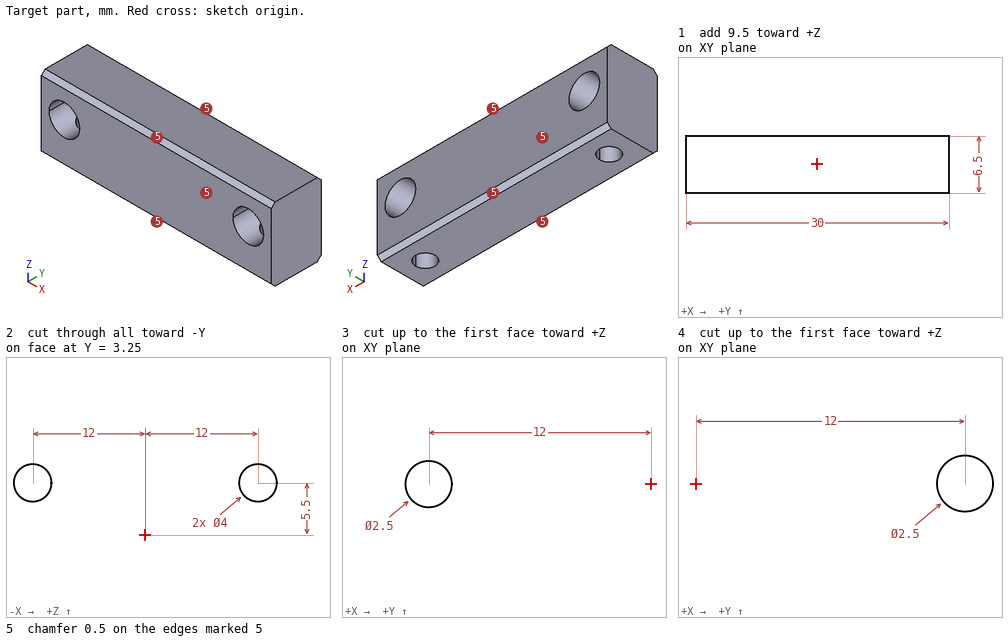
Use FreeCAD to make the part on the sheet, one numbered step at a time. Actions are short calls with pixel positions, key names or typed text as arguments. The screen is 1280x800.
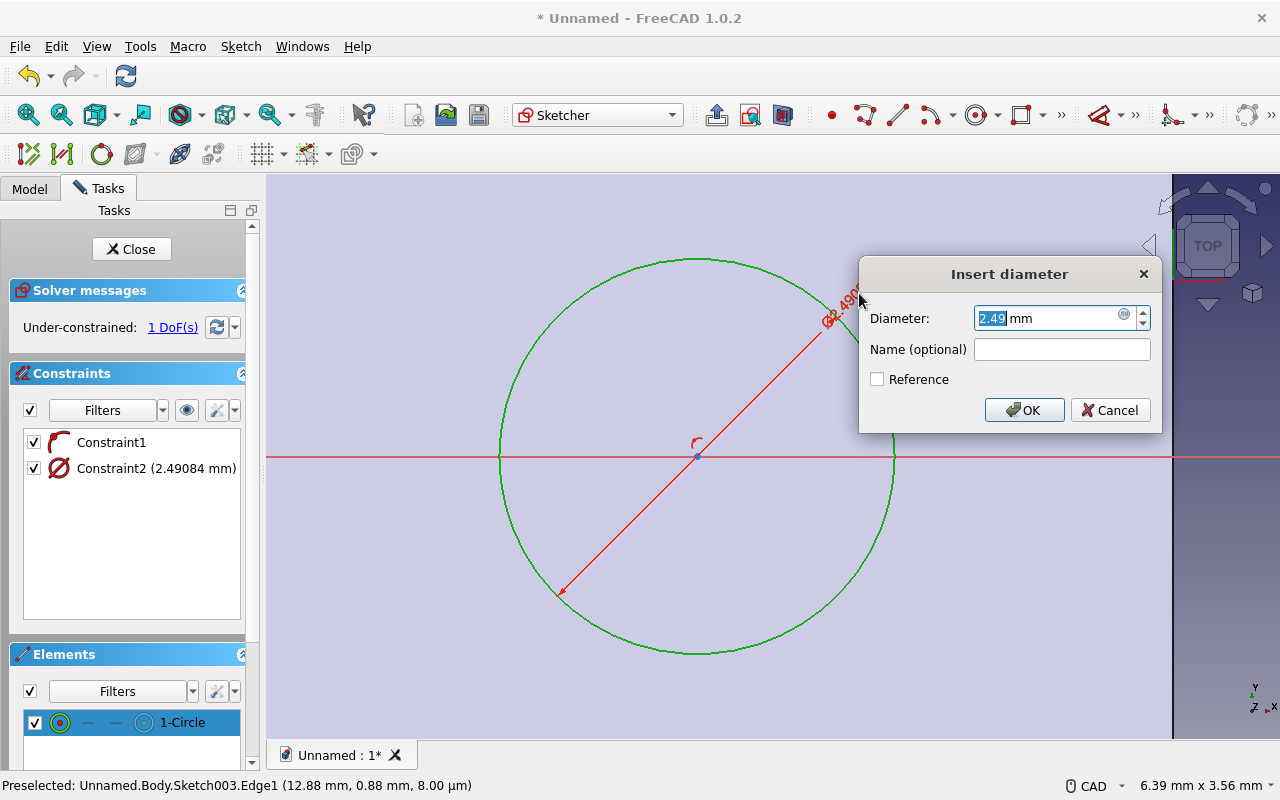
text(2.5)
key(Return)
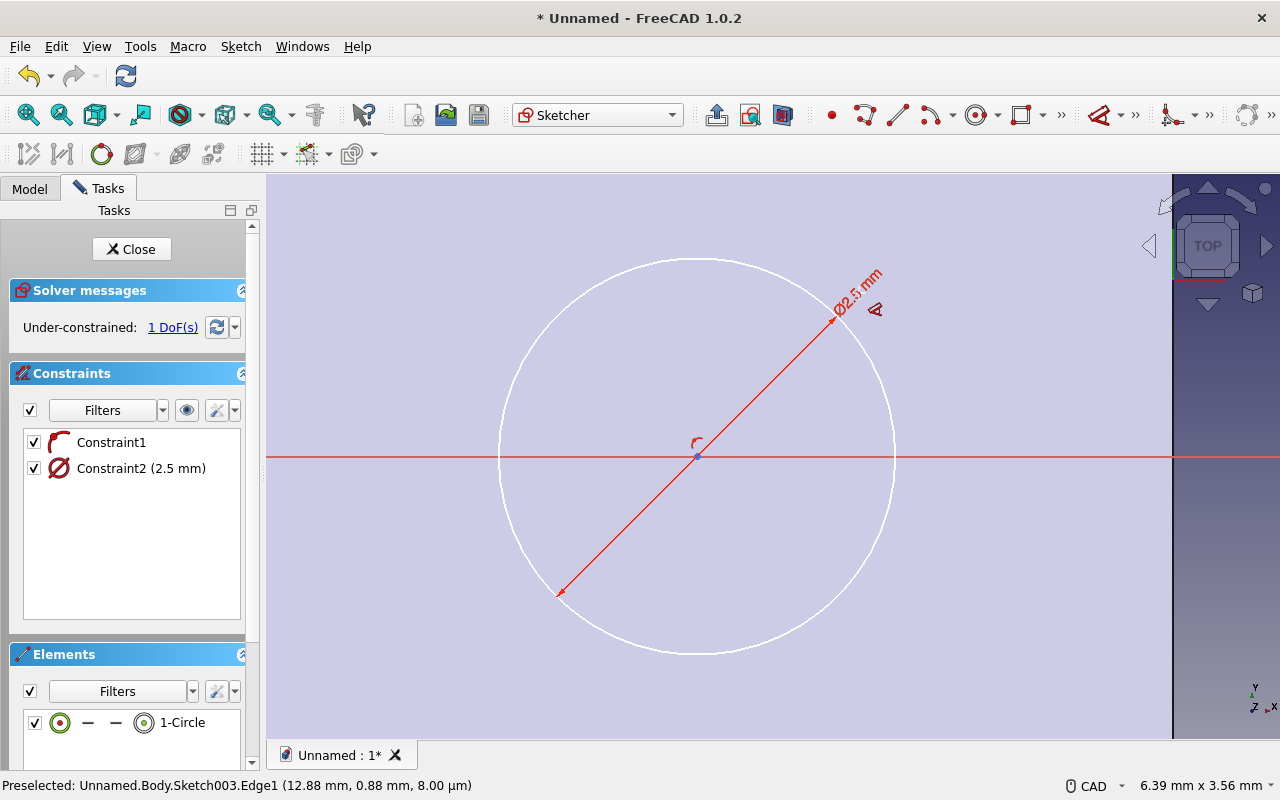
click(697, 456)
click(403, 490)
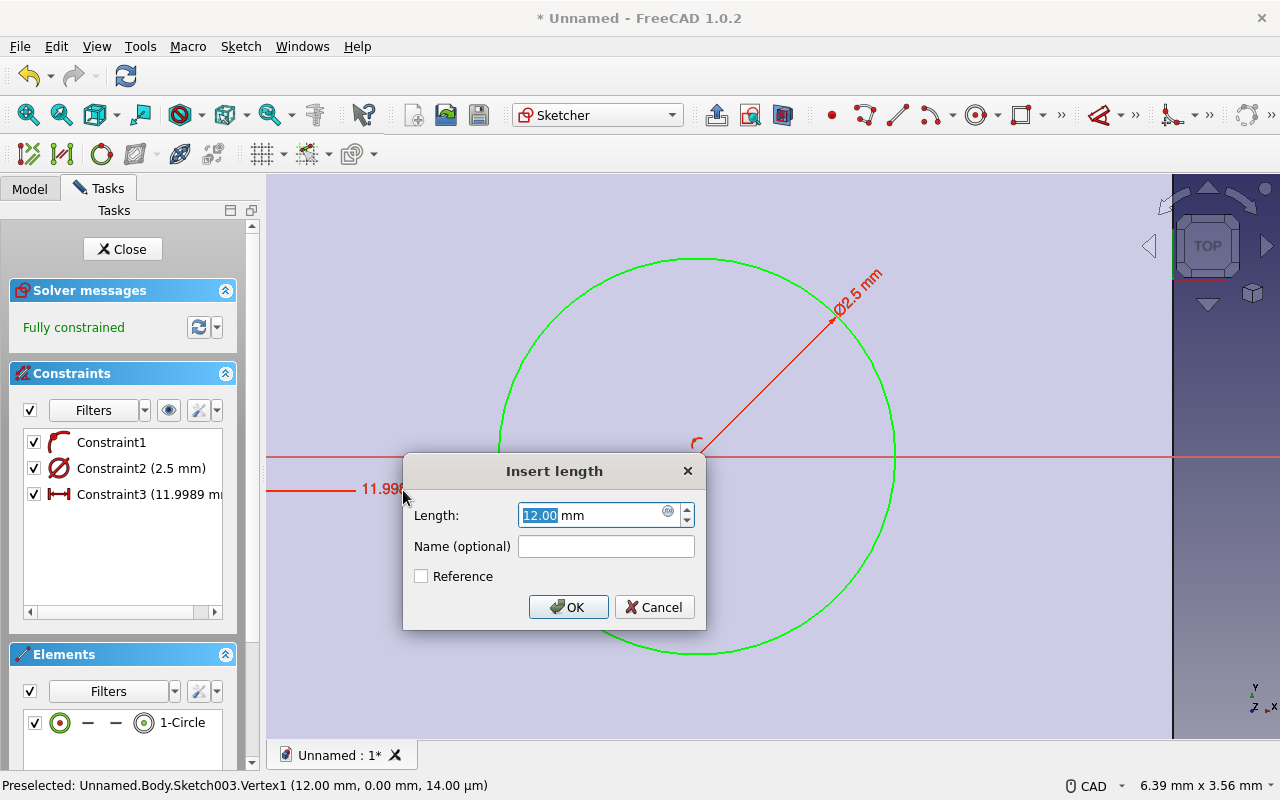
text(12)
key(Return)
key(Escape)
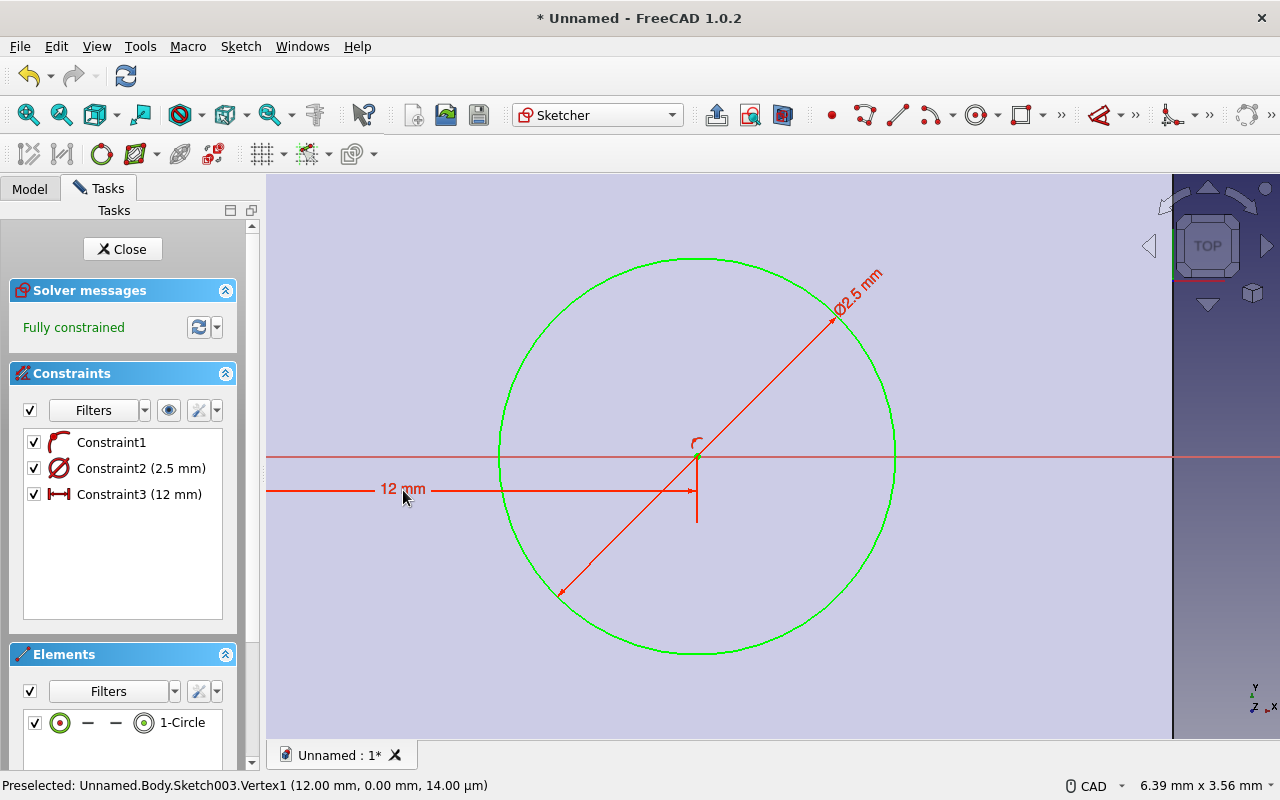
click(123, 249)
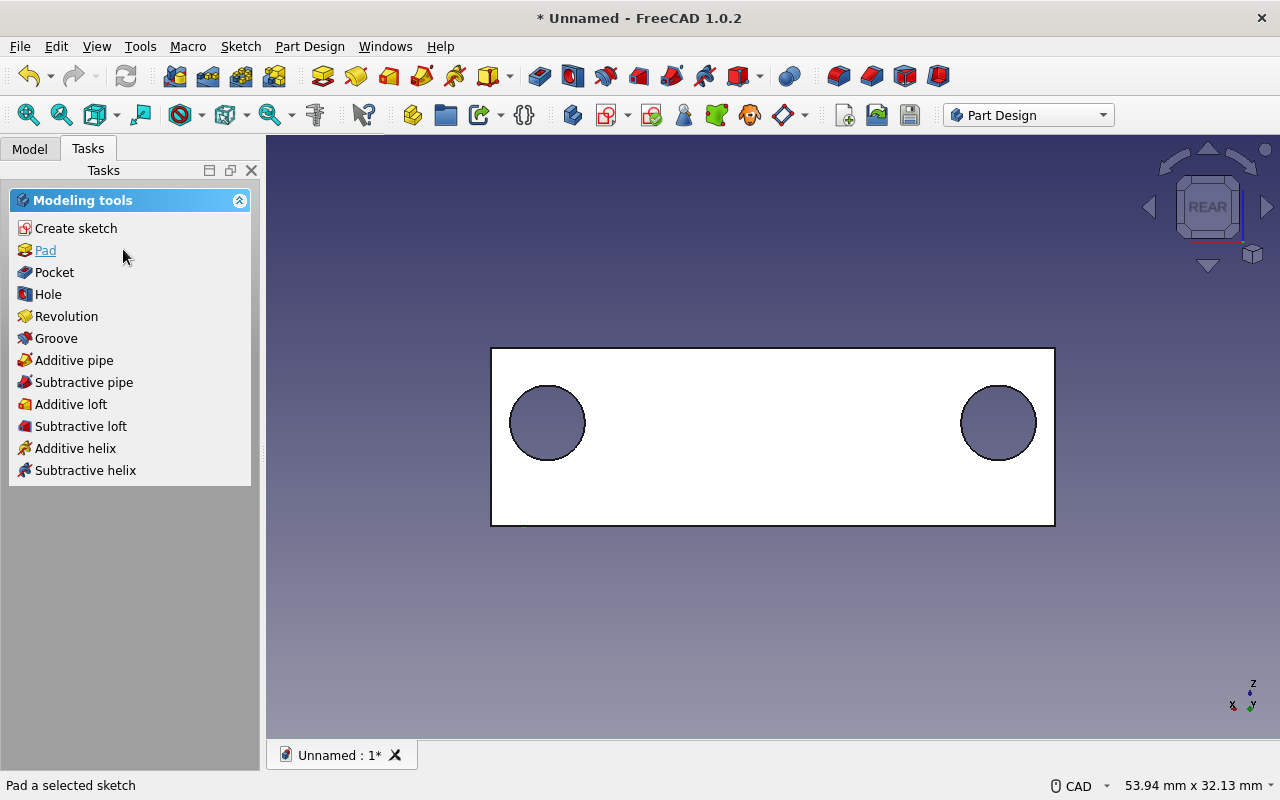
click(540, 76)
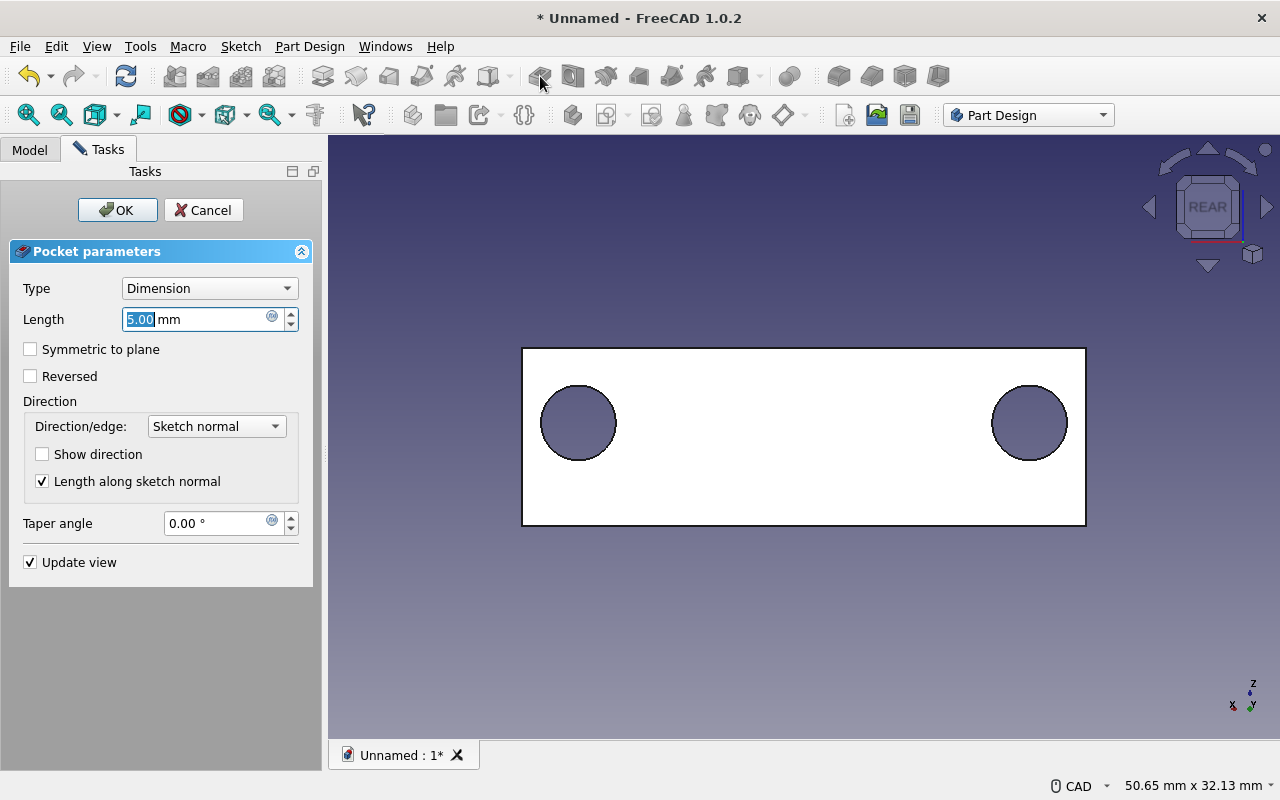
click(210, 288)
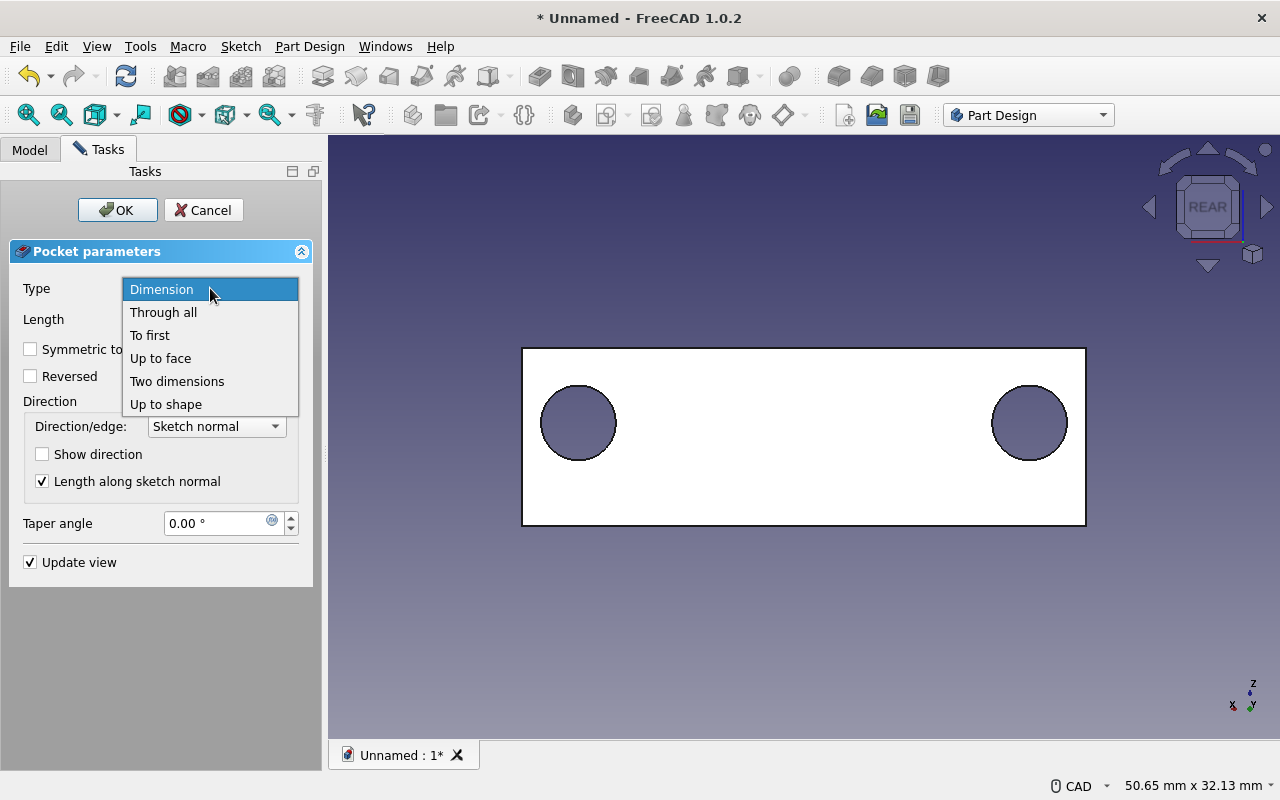
click(208, 336)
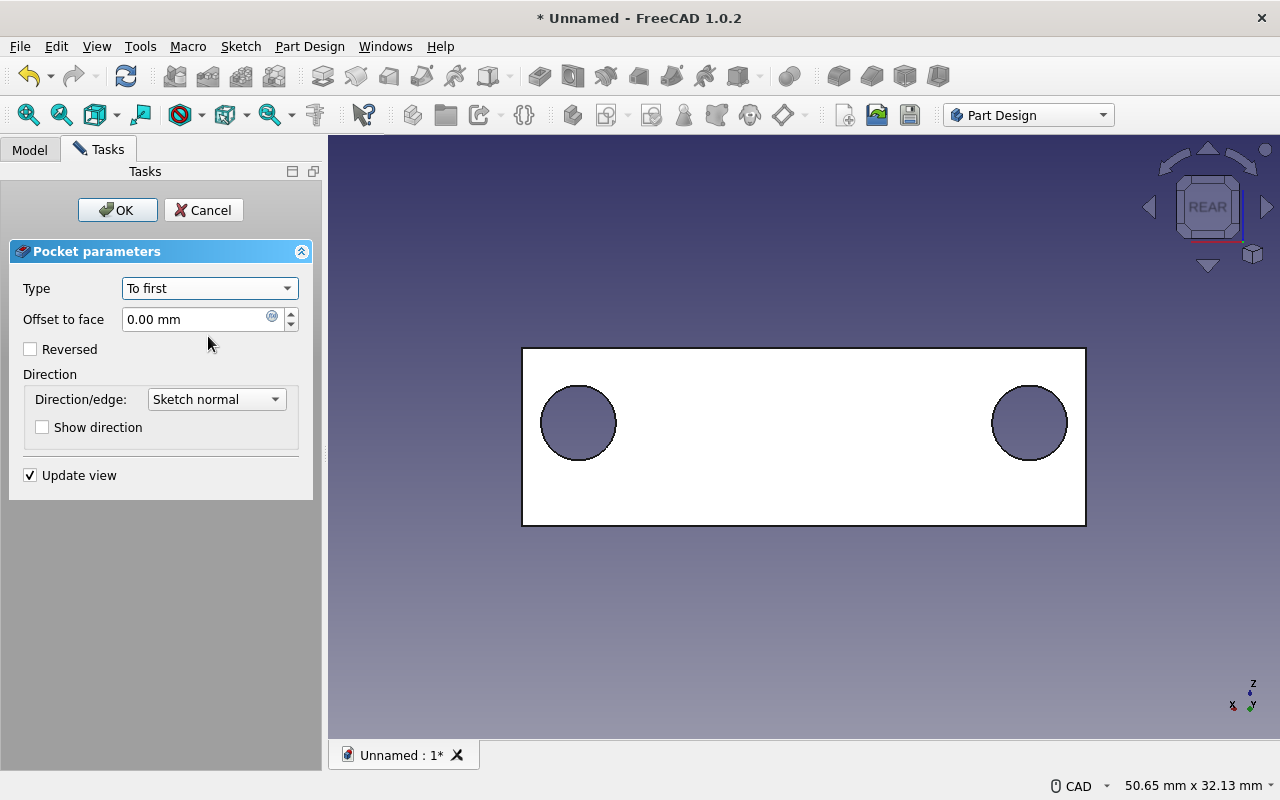
click(31, 349)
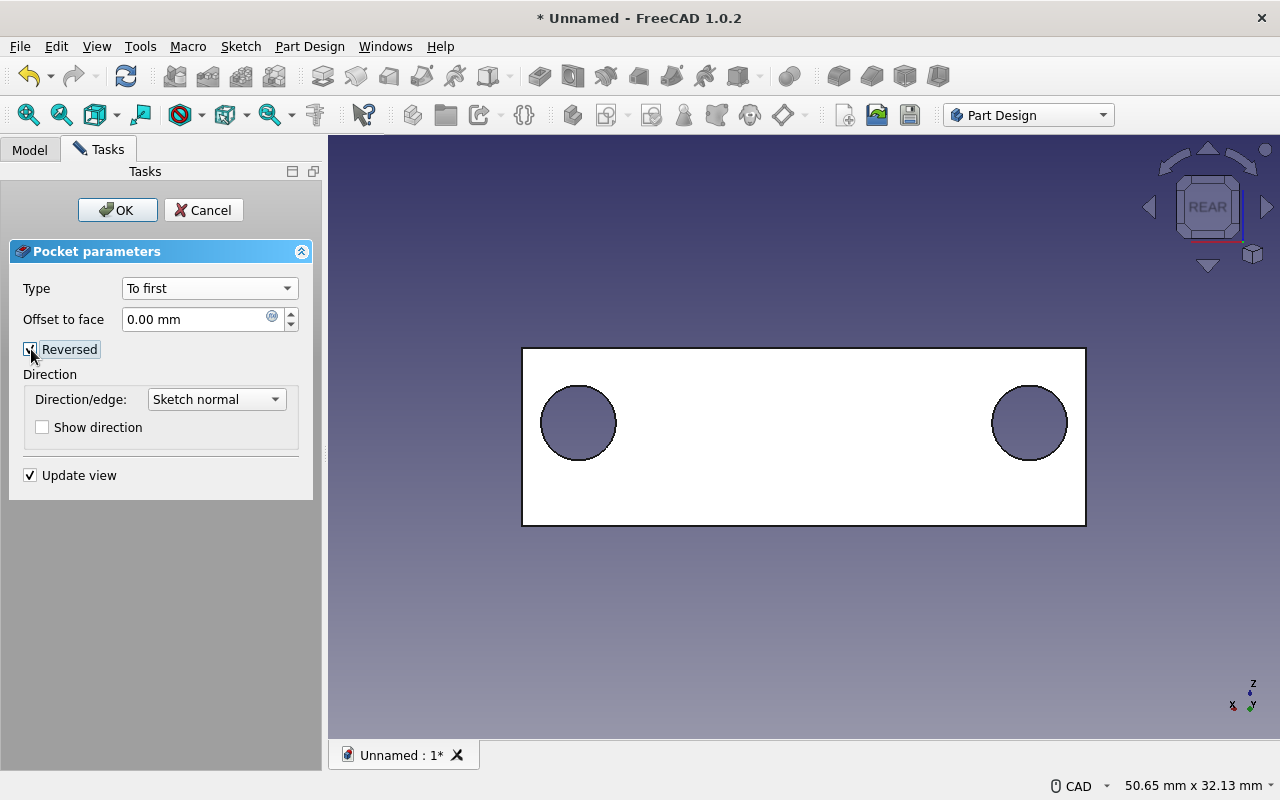
click(118, 210)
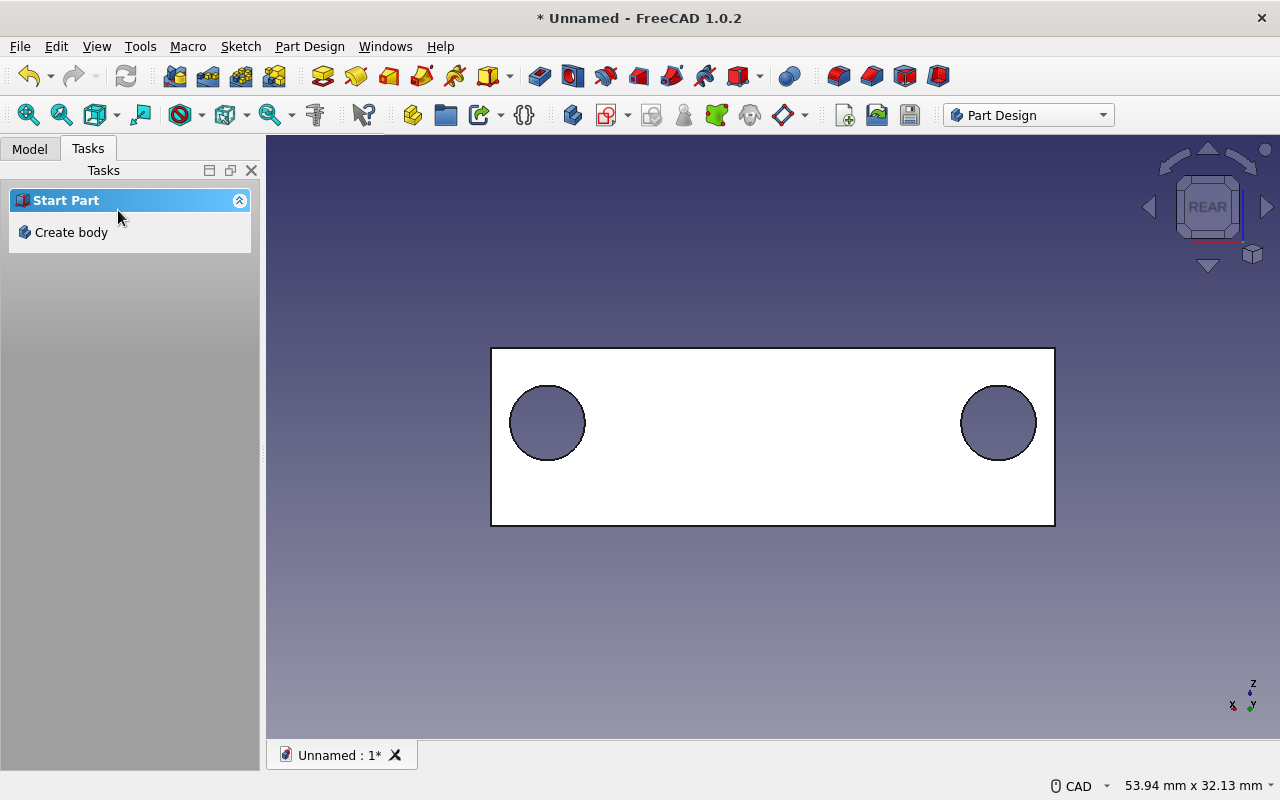
click(773, 347)